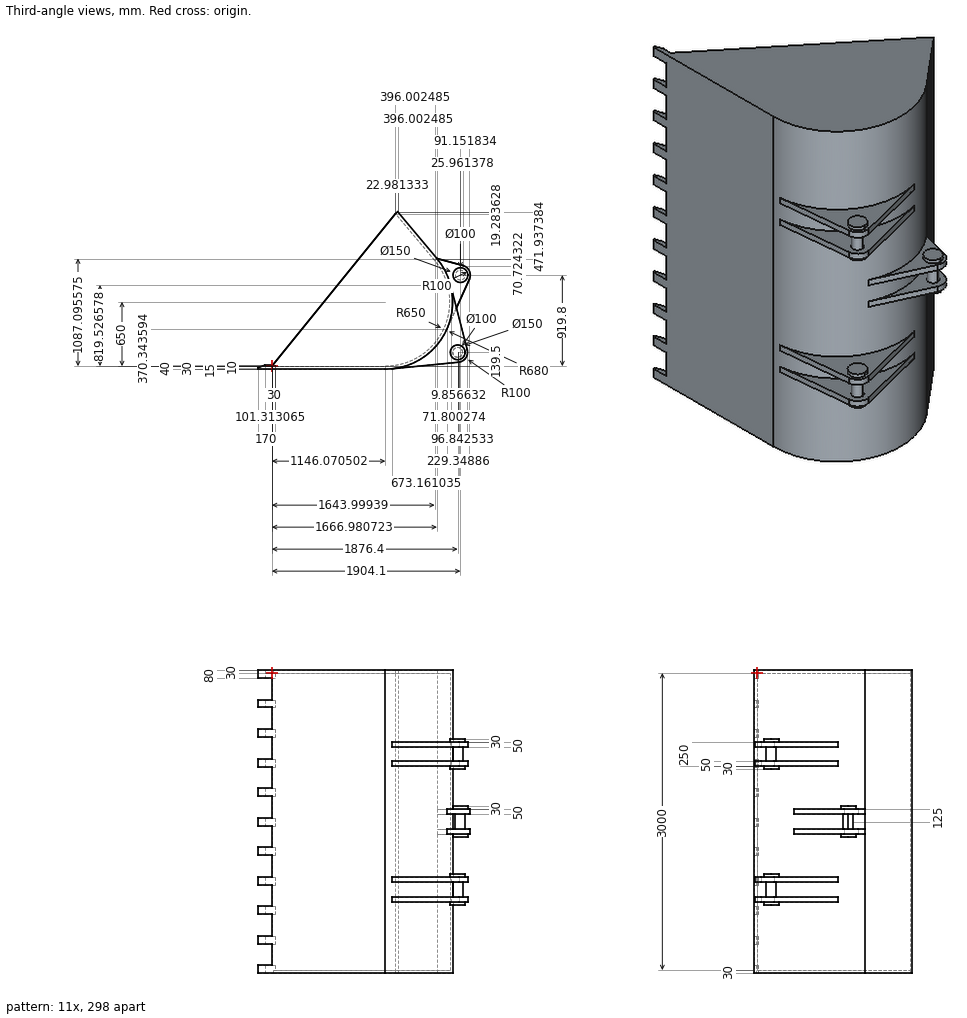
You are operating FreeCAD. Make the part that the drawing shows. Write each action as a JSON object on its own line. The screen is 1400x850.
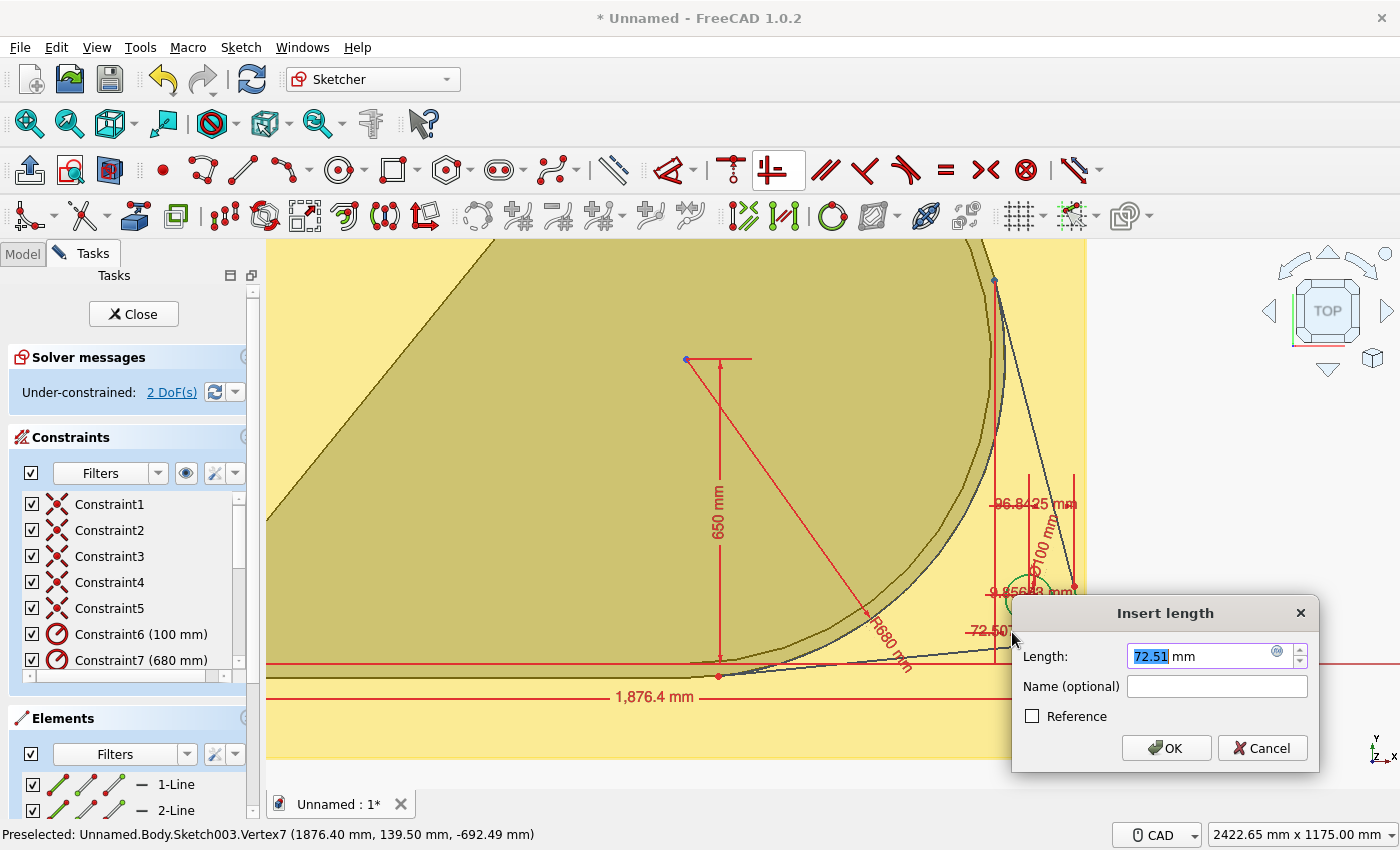
{"action": "type", "text": "71.800274"}
{"action": "key", "text": "Return"}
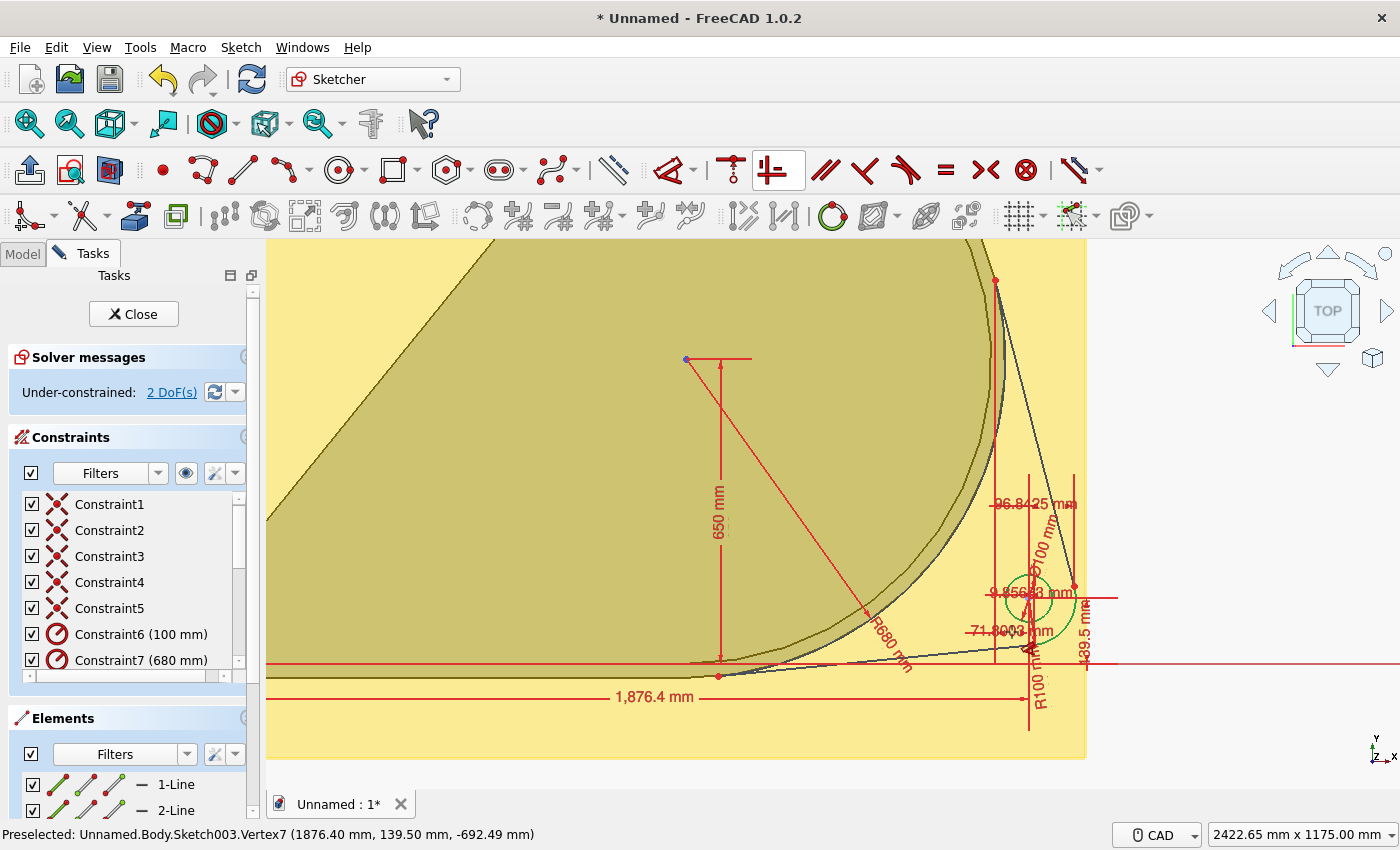
{"action": "left_click", "coordinate": [995, 281]}
{"action": "left_click", "coordinate": [1029, 472]}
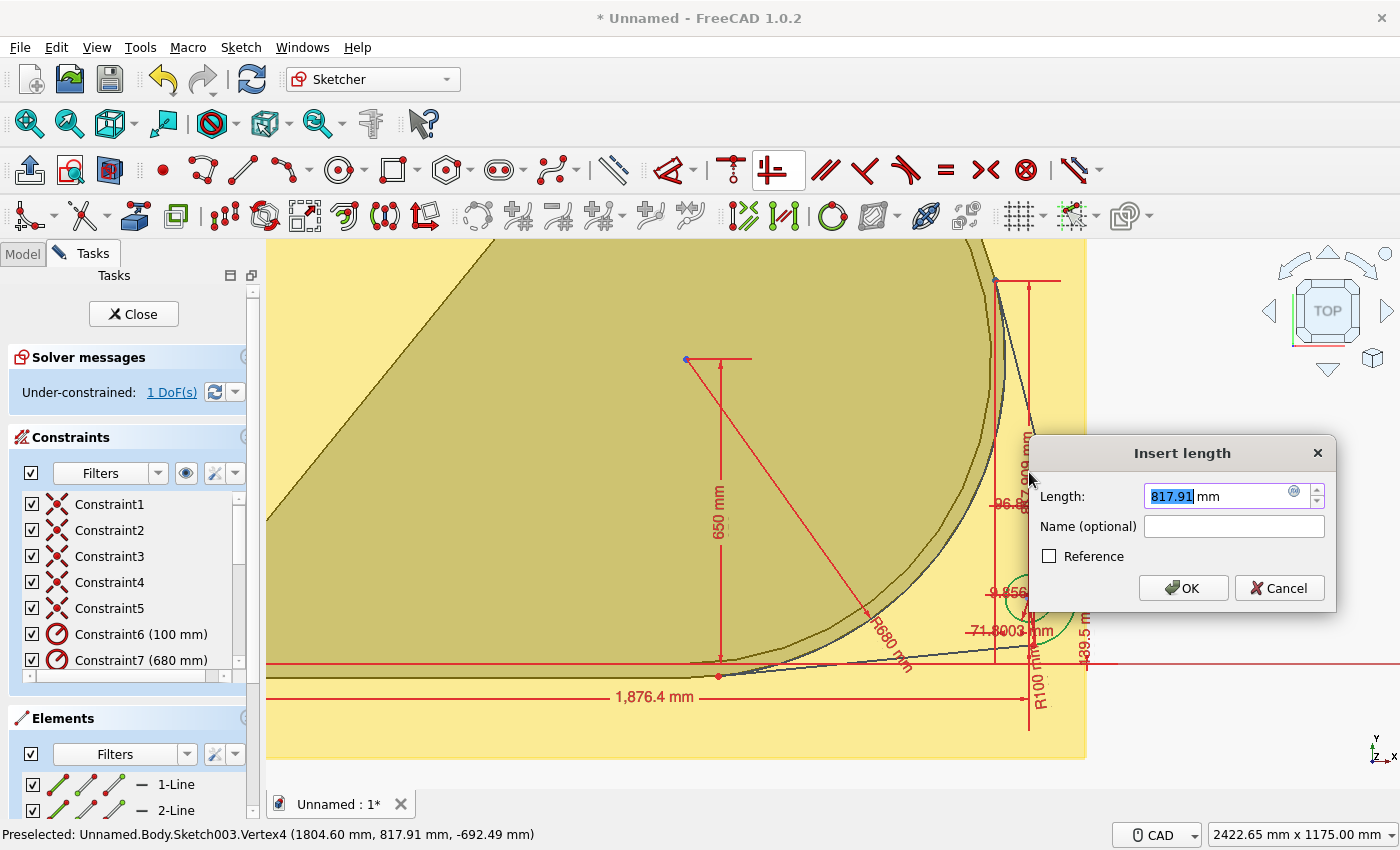
{"action": "type", "text": "819.526578"}
{"action": "key", "text": "Return"}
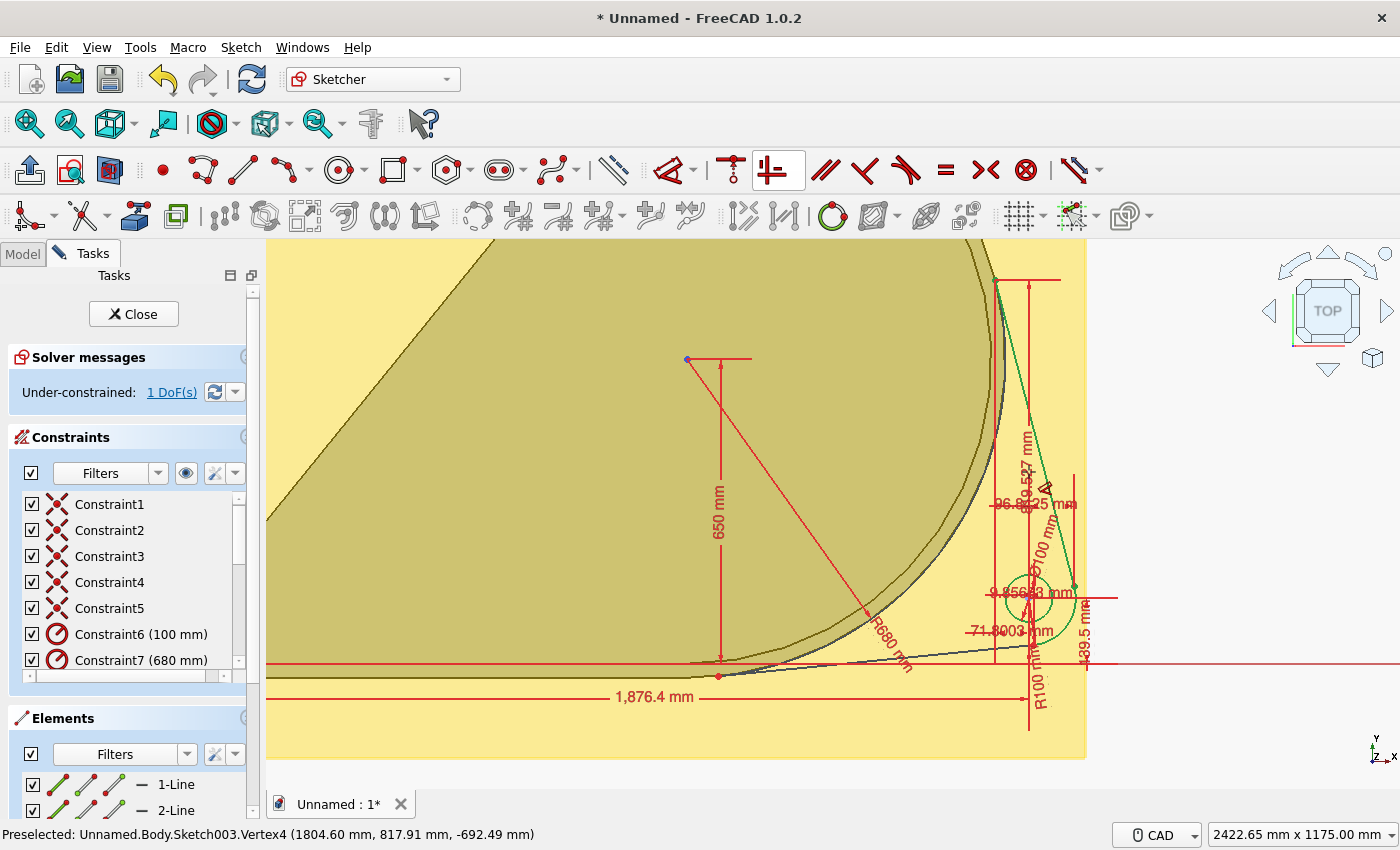
{"action": "left_click", "coordinate": [813, 667]}
{"action": "left_click", "coordinate": [876, 710]}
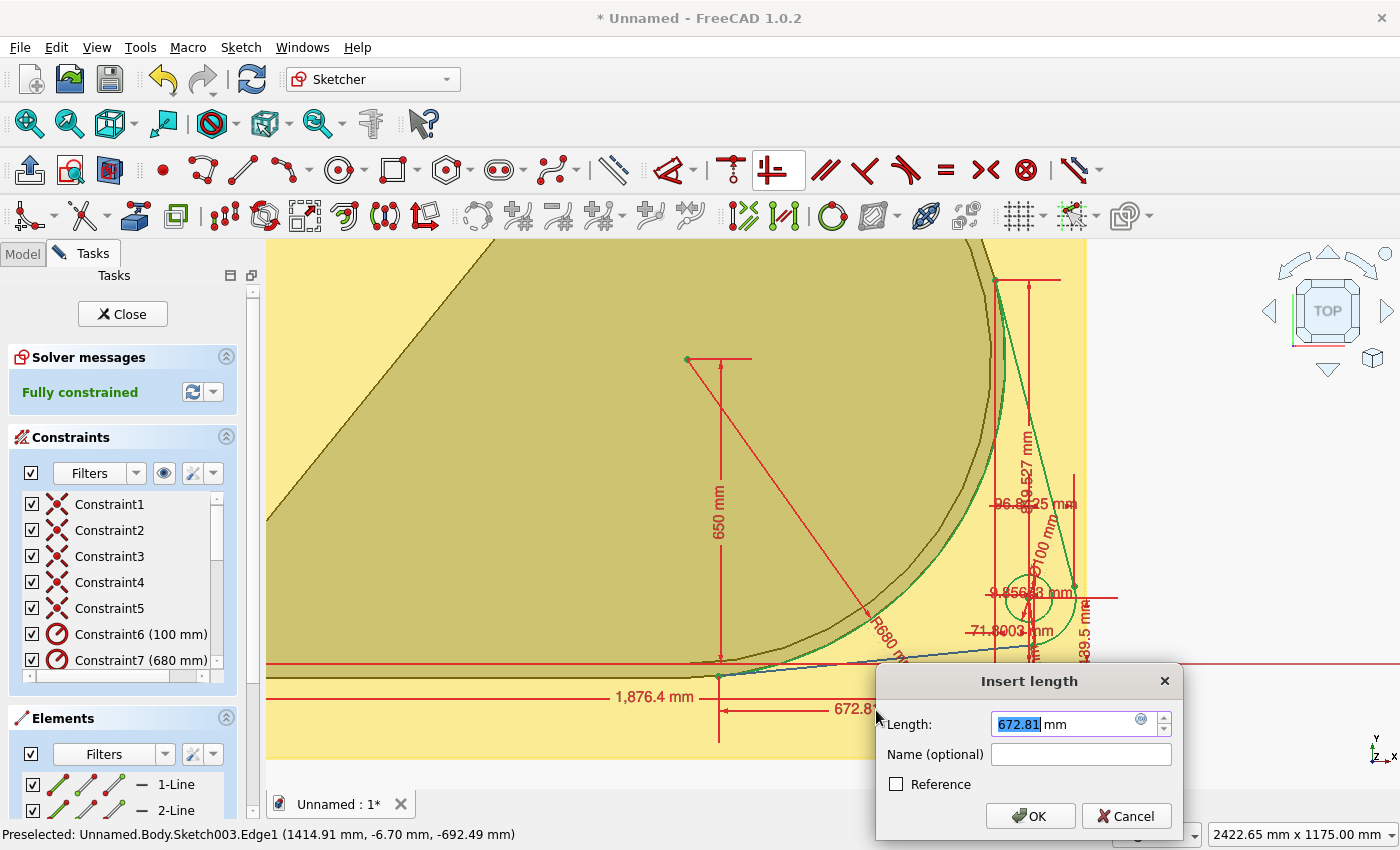
{"action": "type", "text": "673.161035"}
{"action": "key", "text": "Return"}
{"action": "key", "text": "Escape"}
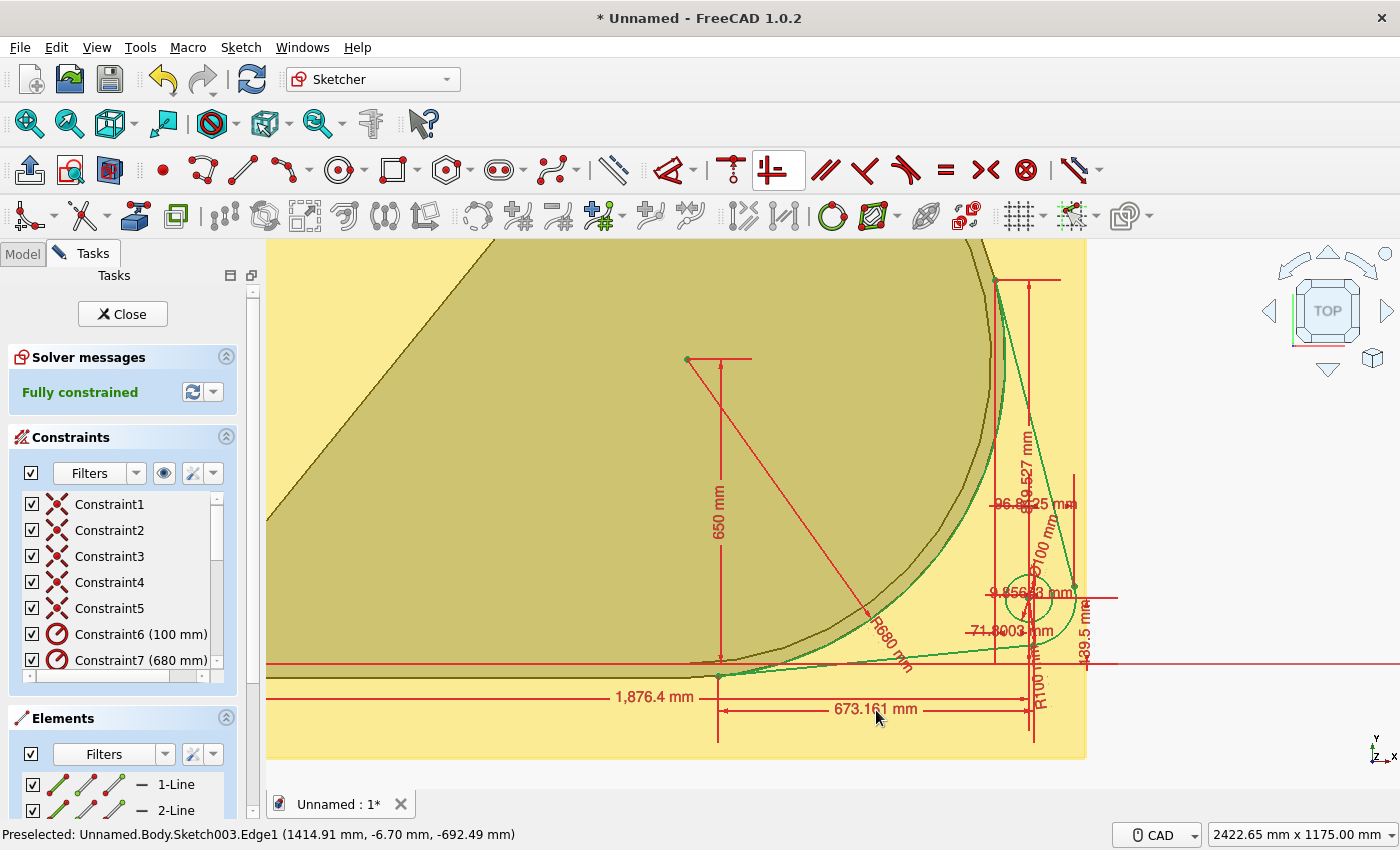
{"action": "left_click", "coordinate": [123, 314]}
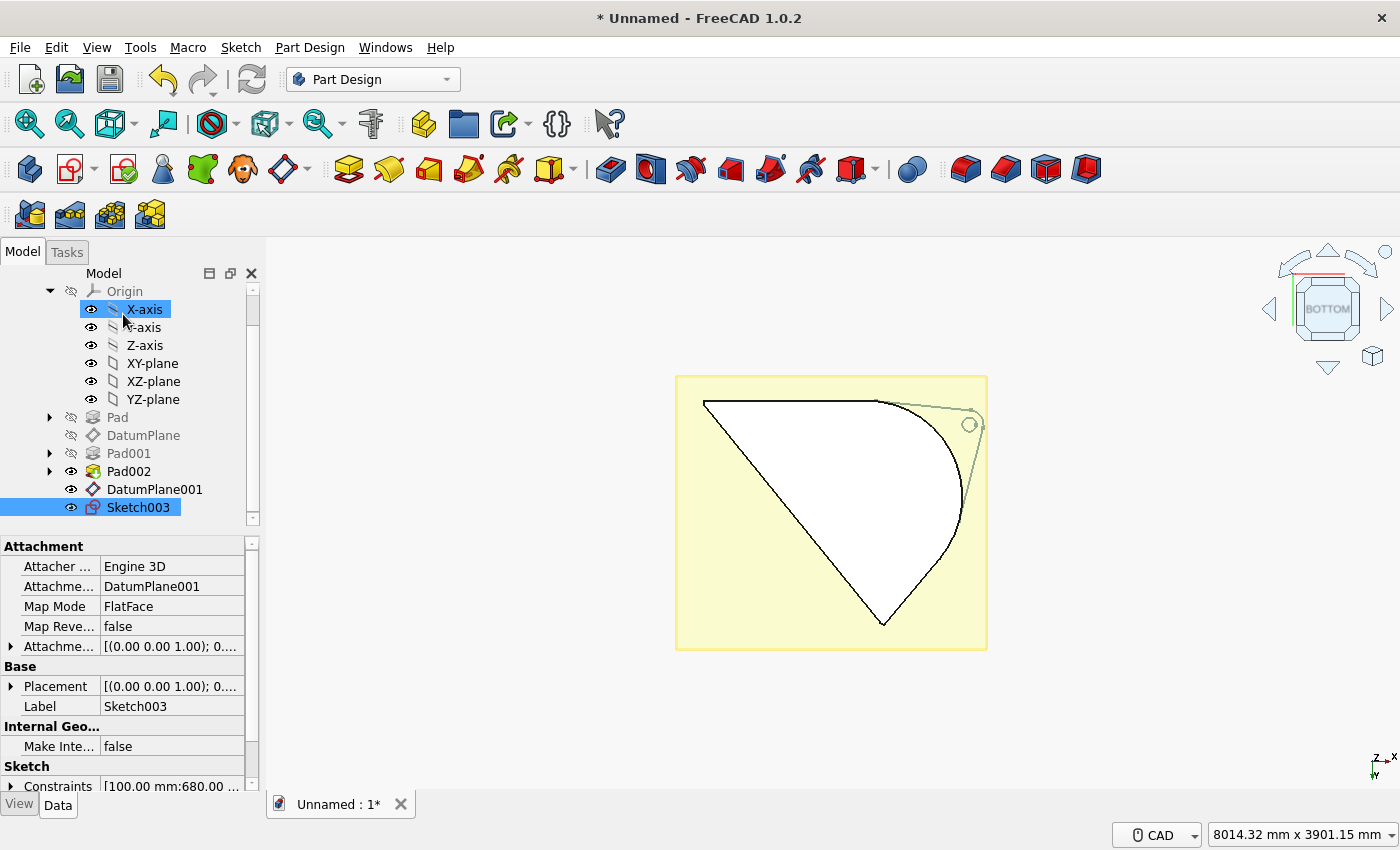
{"action": "left_click", "coordinate": [350, 170]}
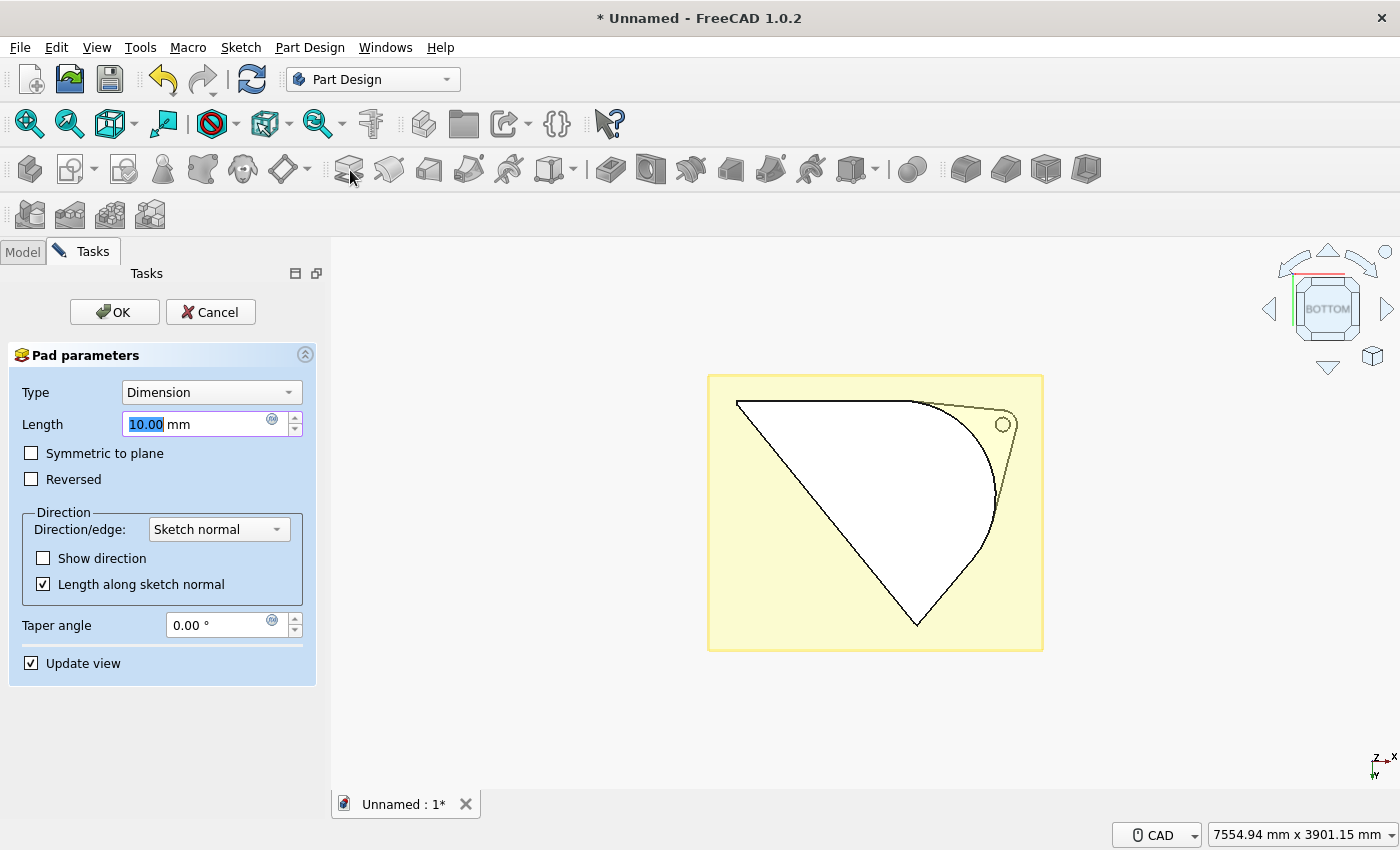
{"action": "type", "text": "50"}
{"action": "key", "text": "Tab"}